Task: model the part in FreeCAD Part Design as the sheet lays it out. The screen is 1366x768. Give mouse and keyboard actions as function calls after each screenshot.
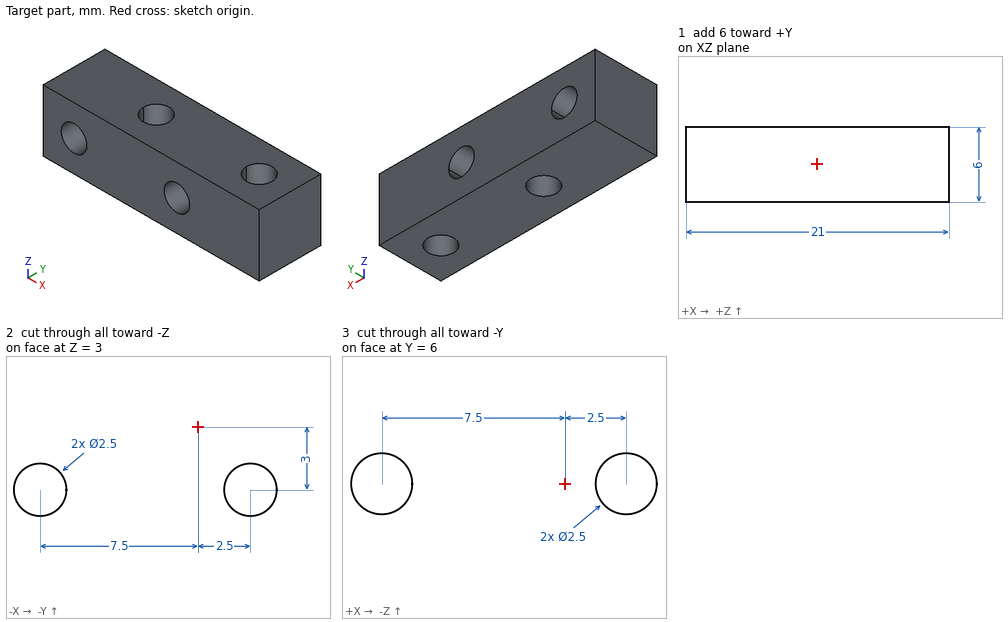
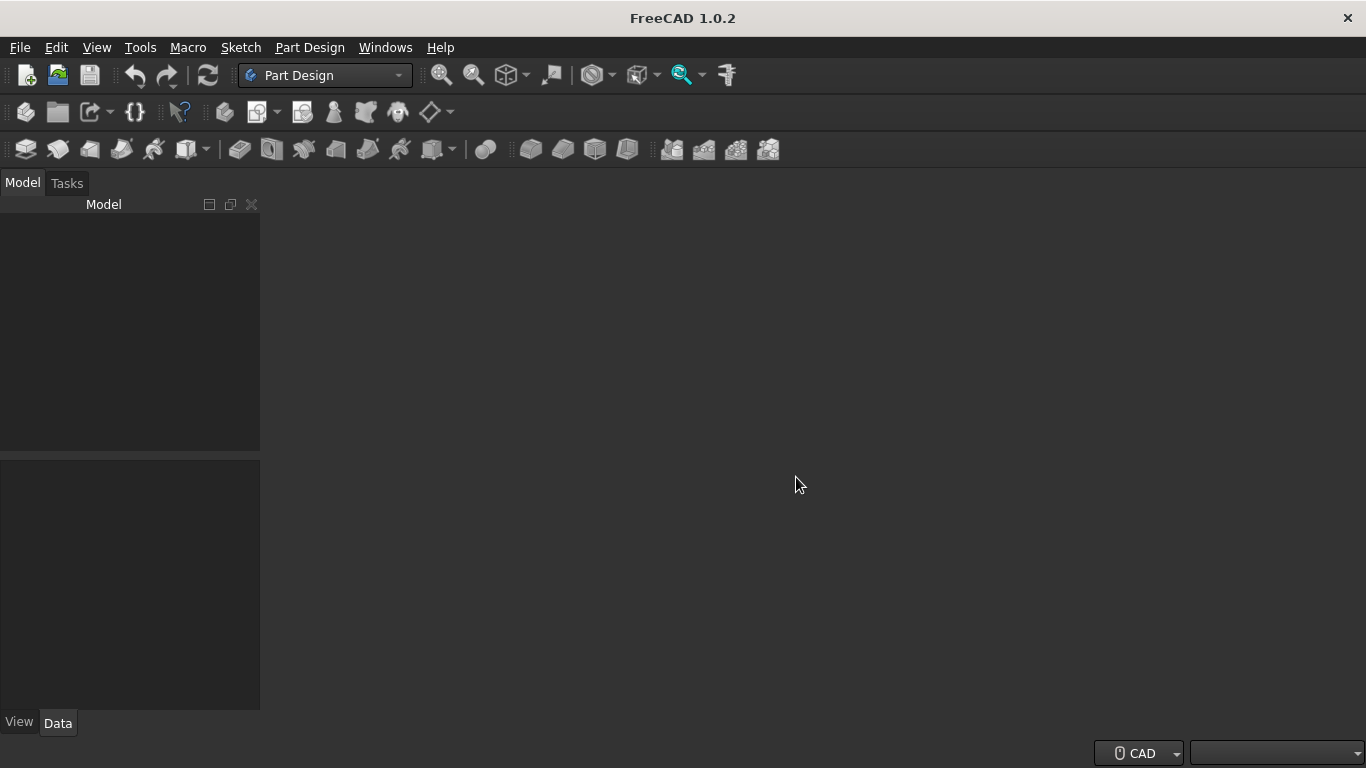
click(26, 76)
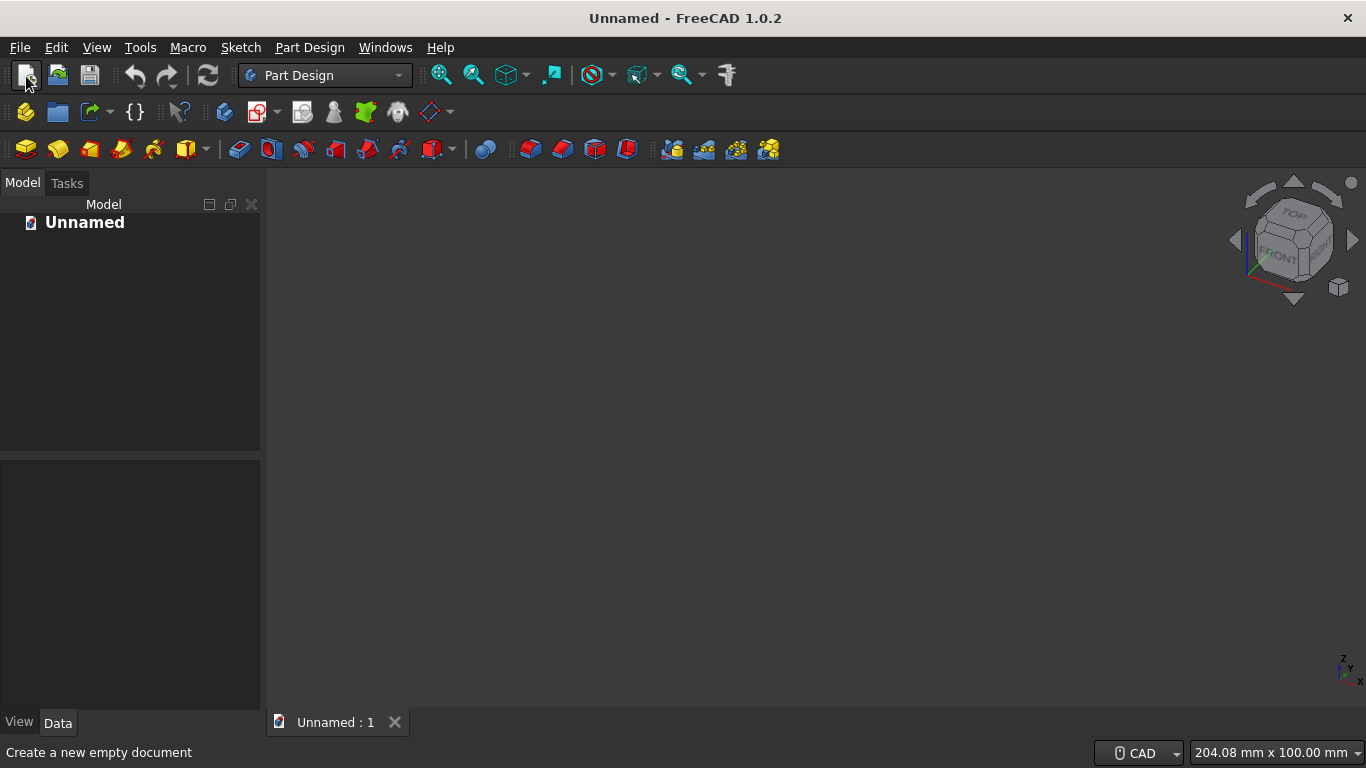
click(258, 112)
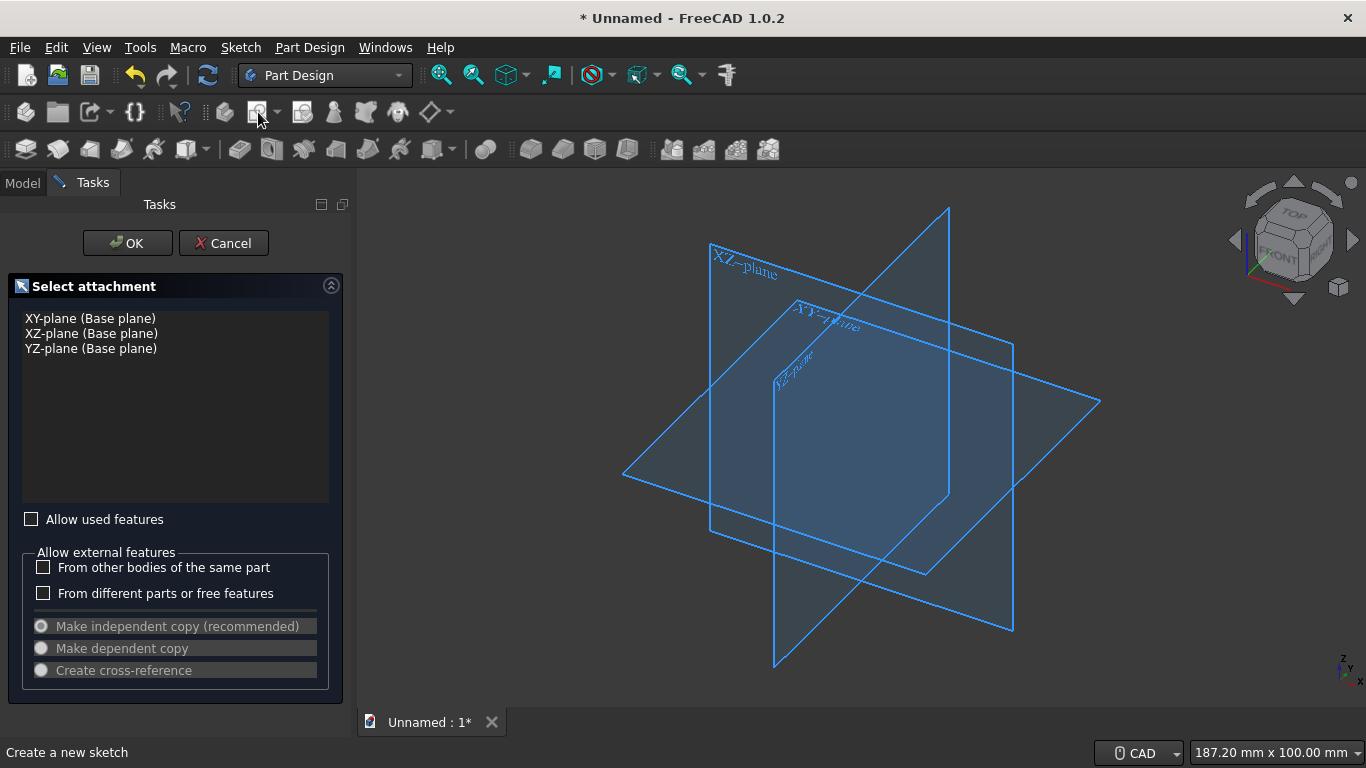
click(82, 334)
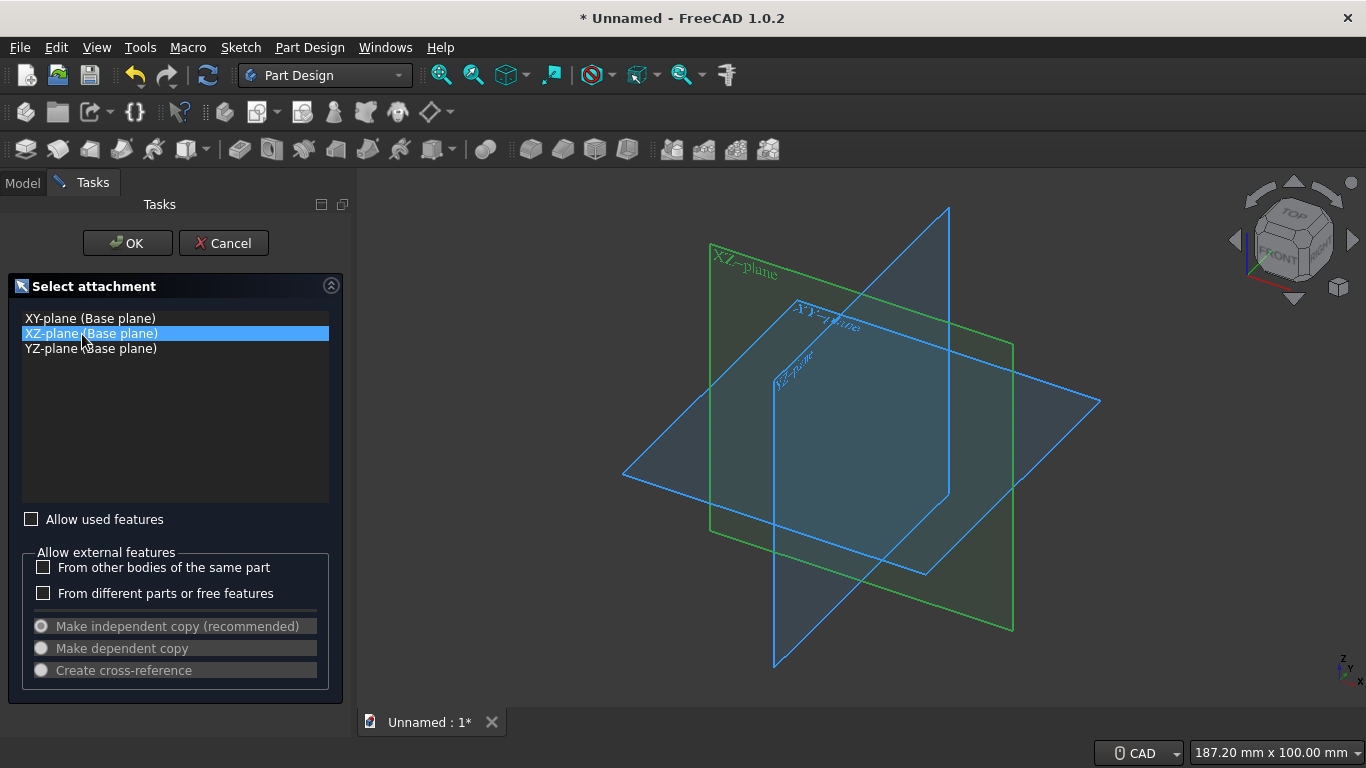
click(128, 243)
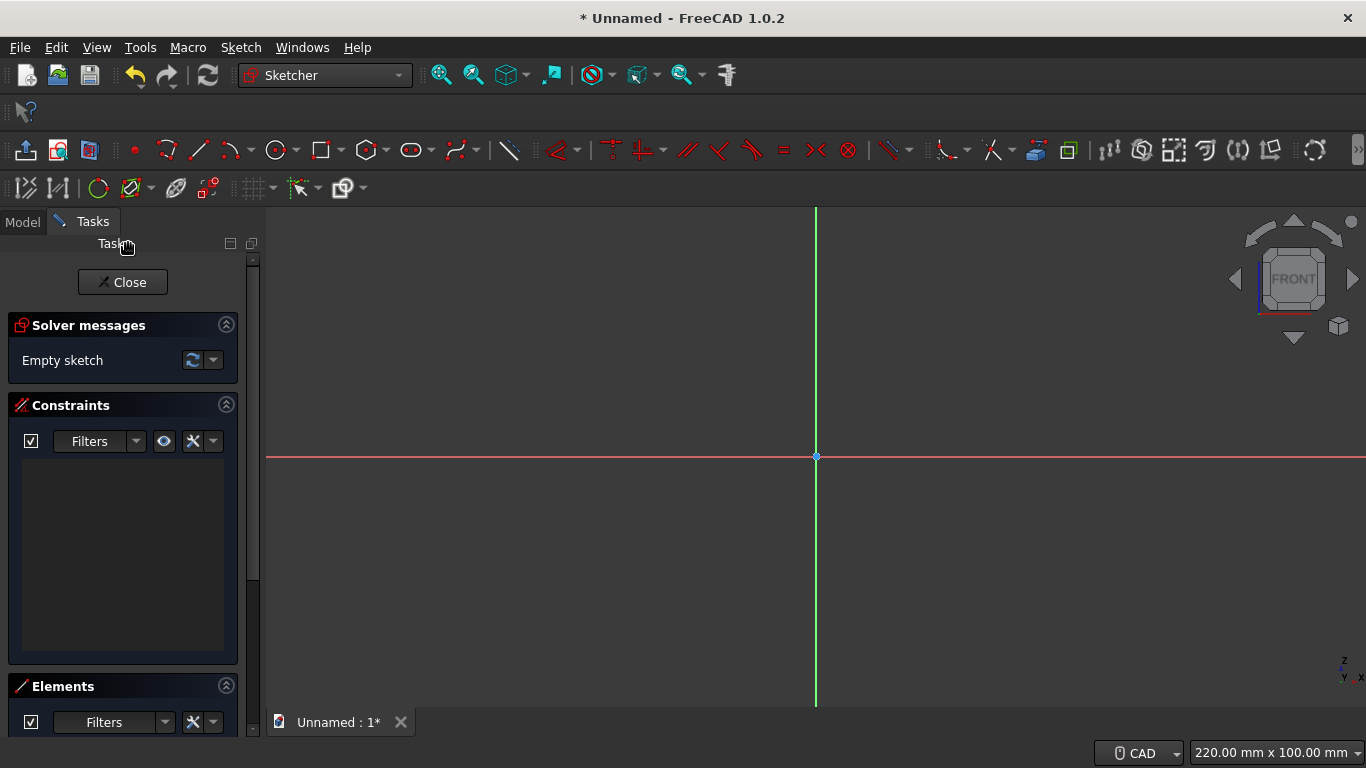
scroll(830, 457, up, 9)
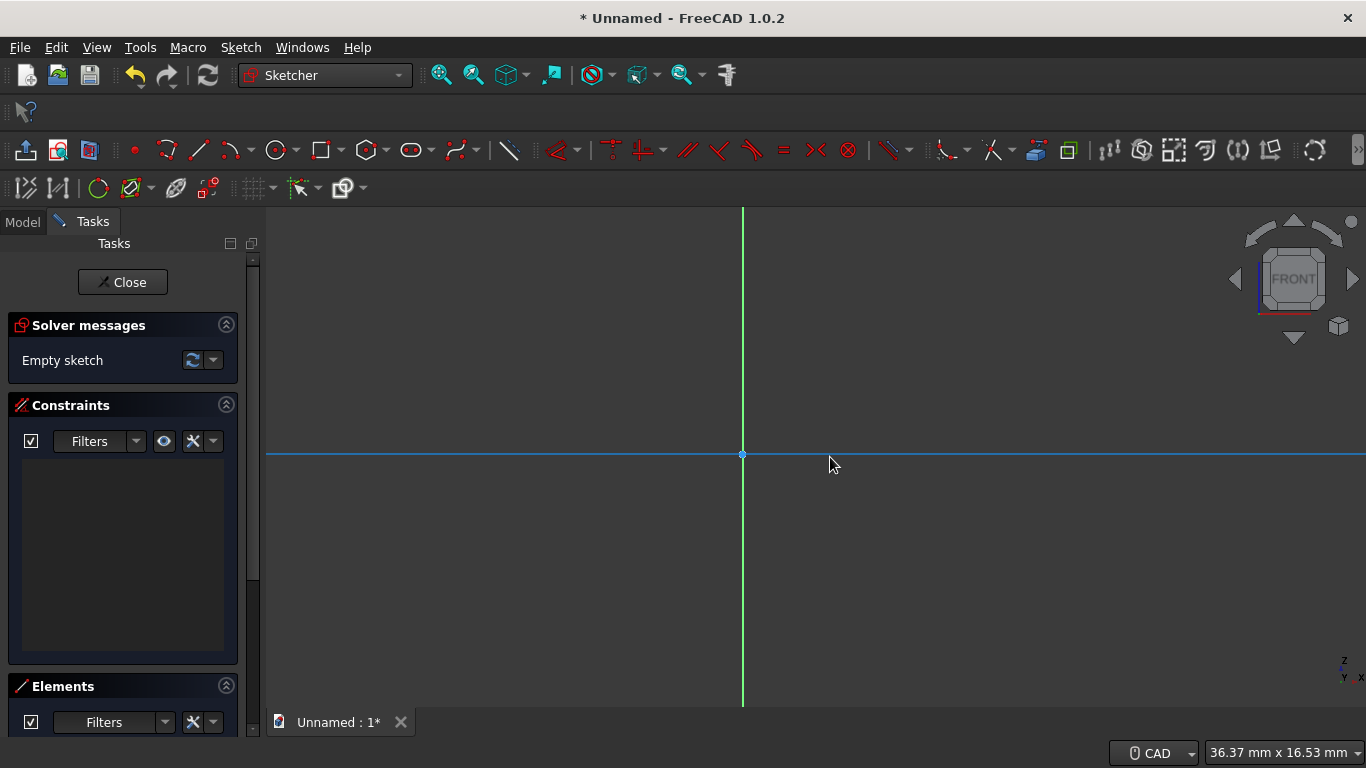
click(344, 150)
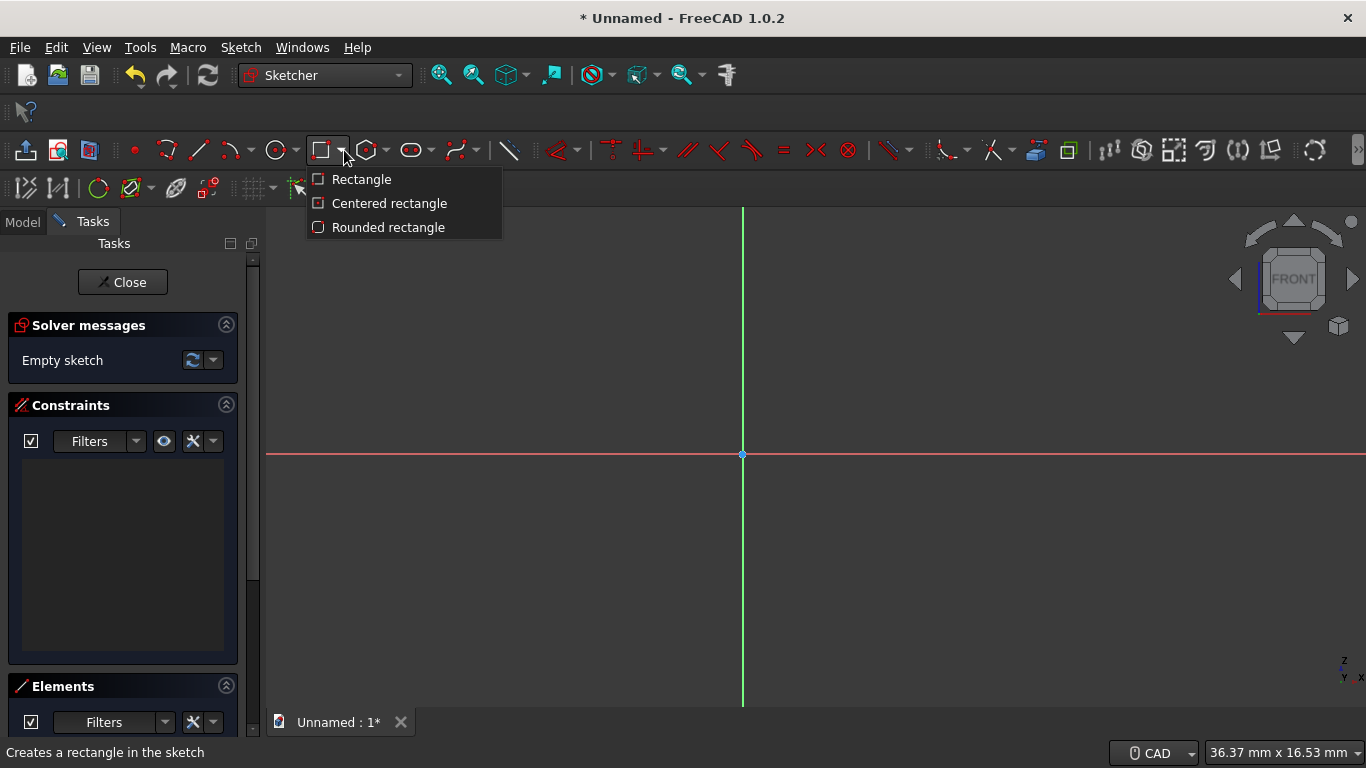
click(404, 203)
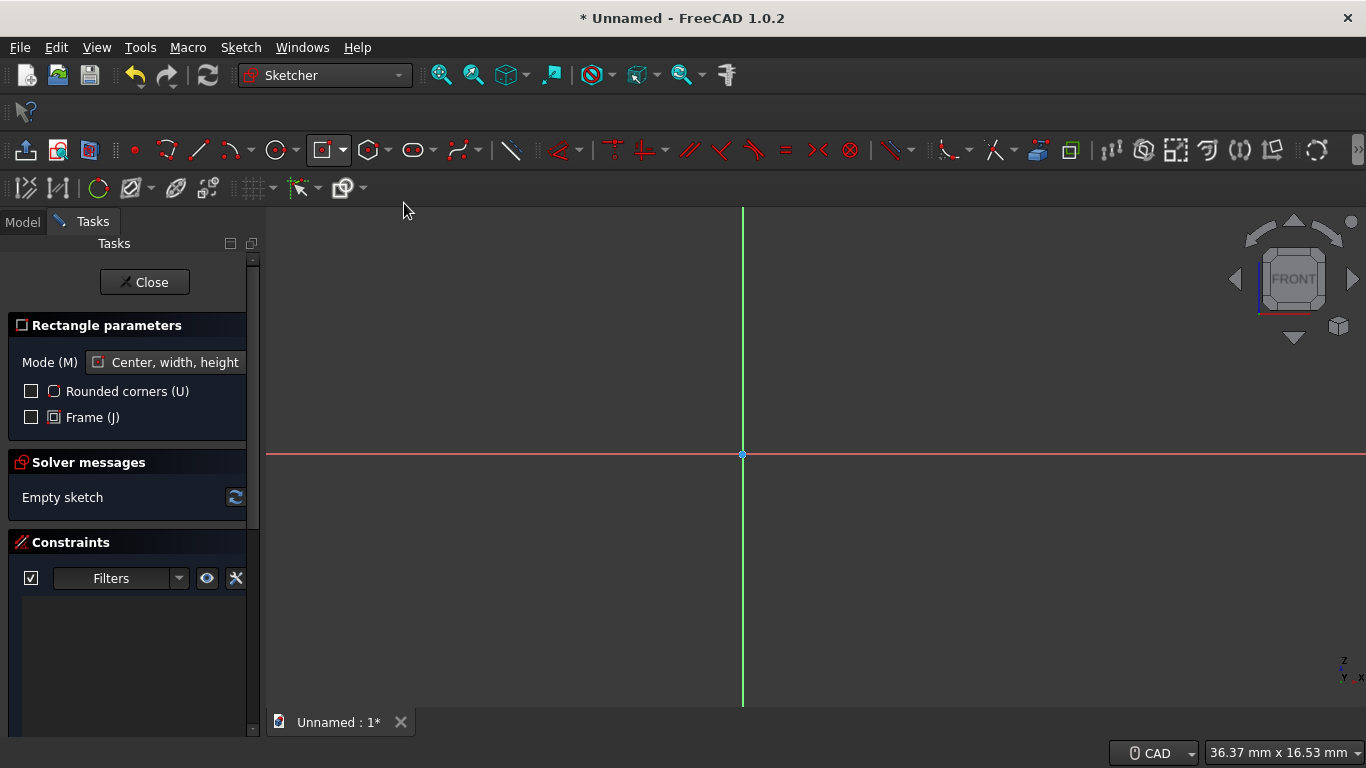
click(743, 454)
move(1060, 364)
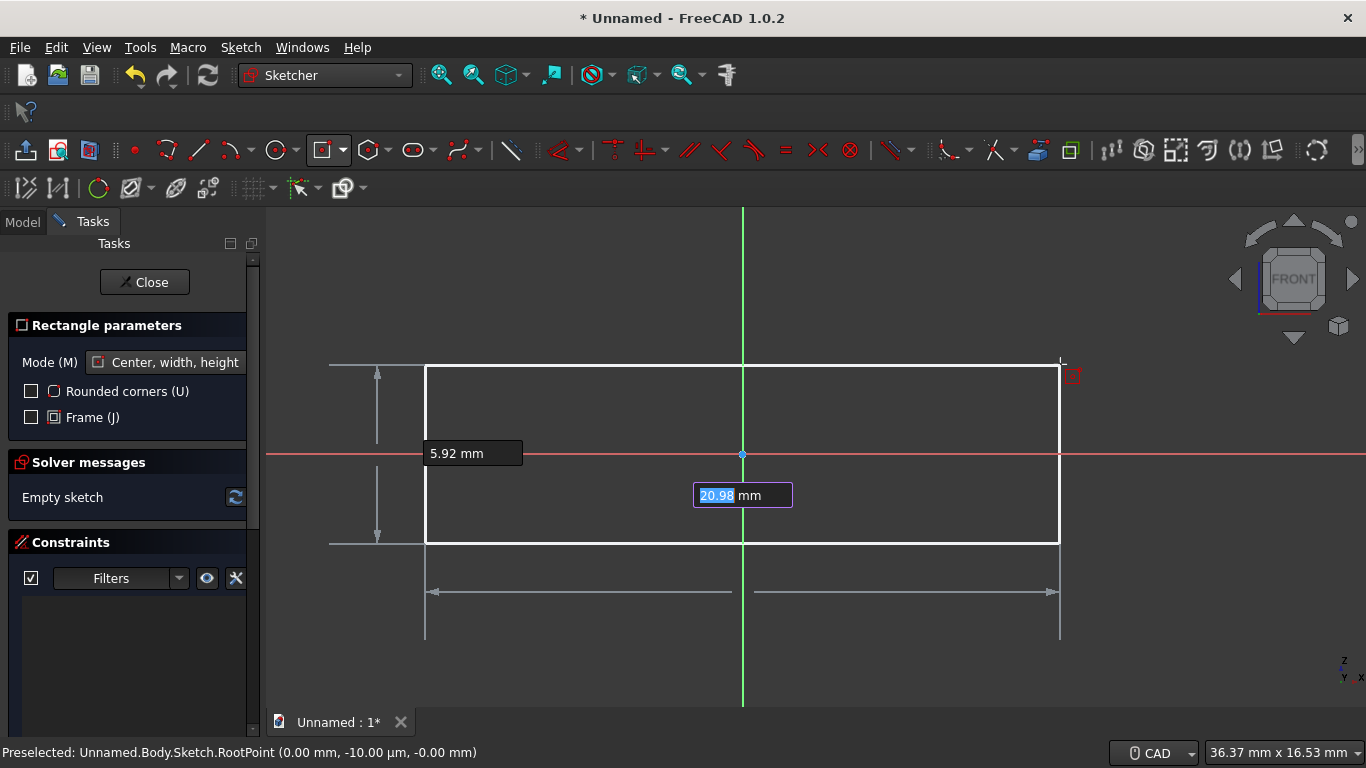
text(21)
key(Tab)
text(6)
key(Return)
key(Escape)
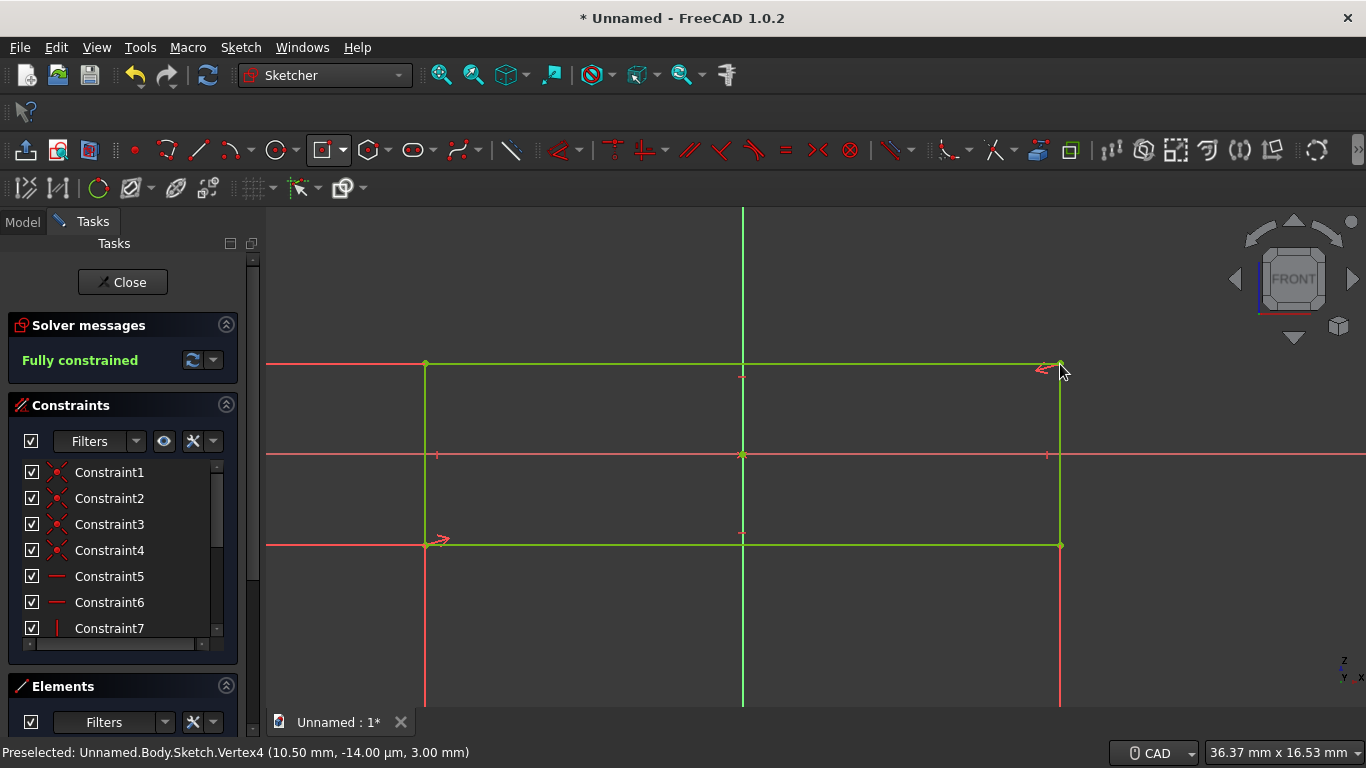
click(123, 282)